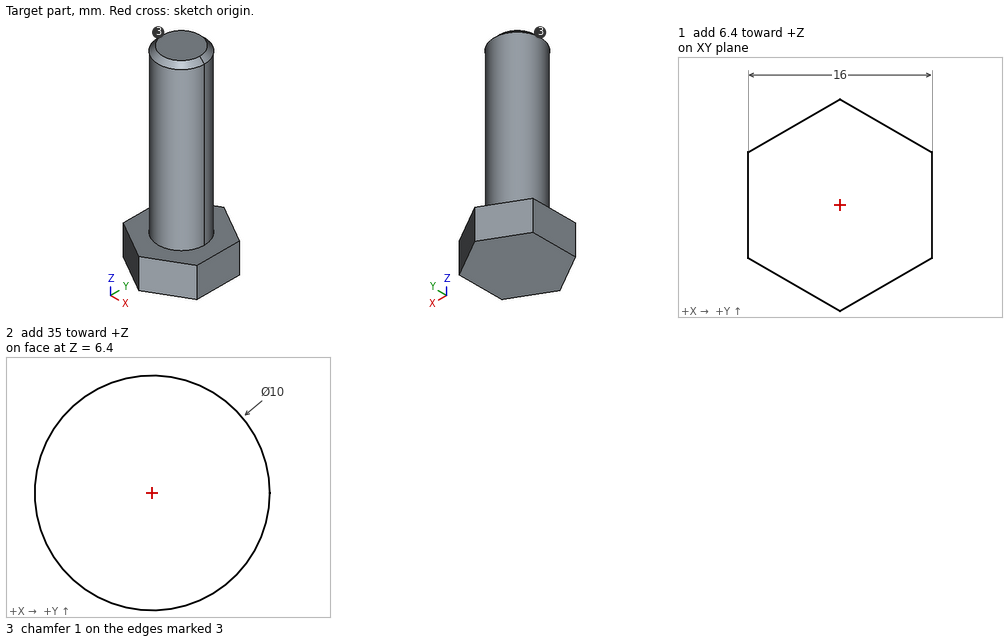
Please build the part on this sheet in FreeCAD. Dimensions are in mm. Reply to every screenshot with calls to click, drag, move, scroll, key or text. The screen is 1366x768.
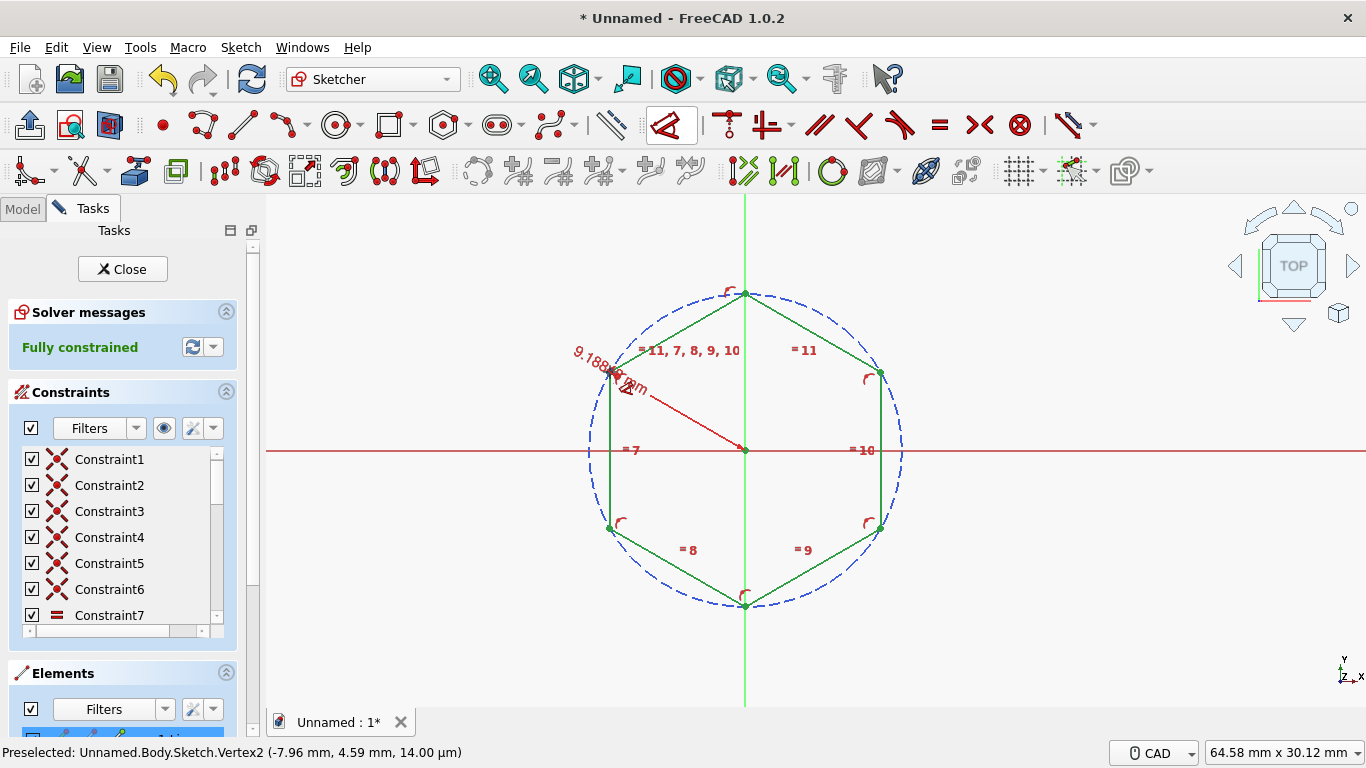
click(881, 529)
click(683, 611)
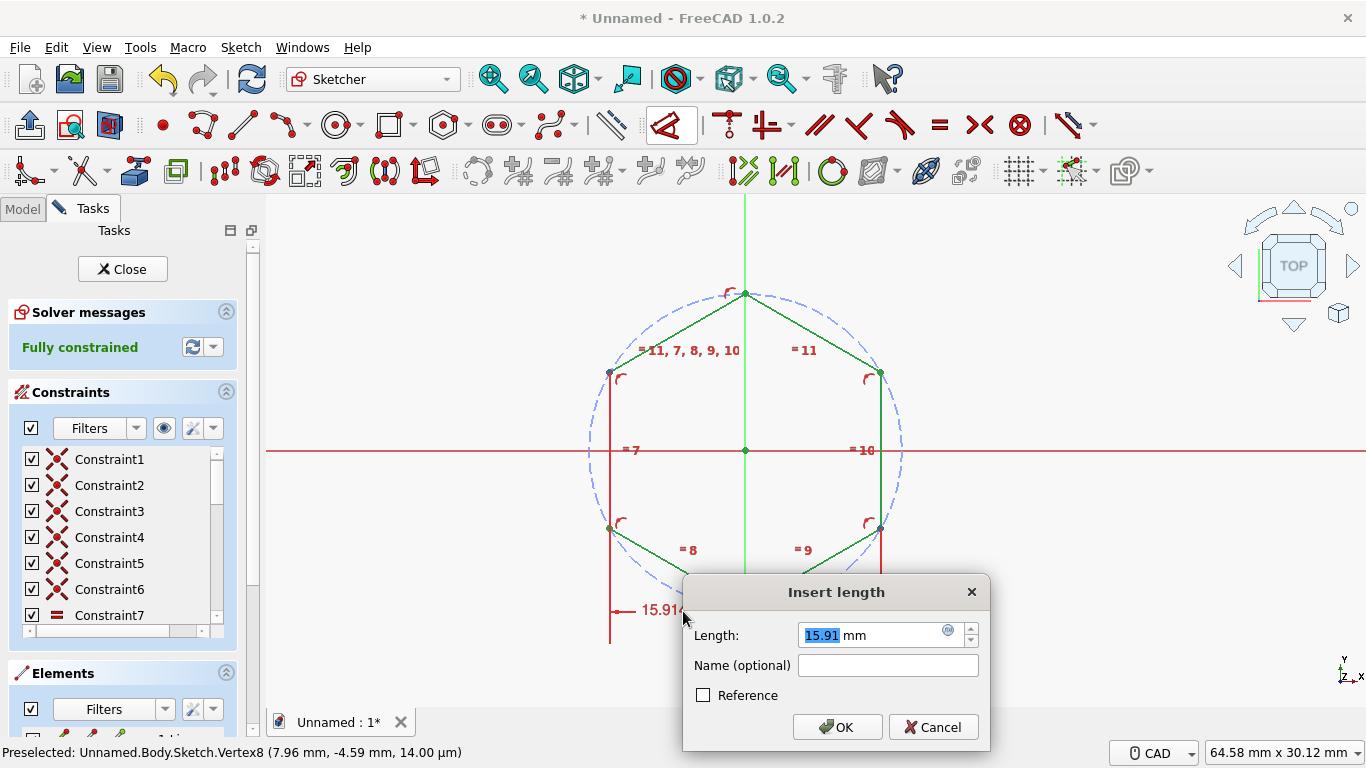
text(16)
key(Return)
key(Escape)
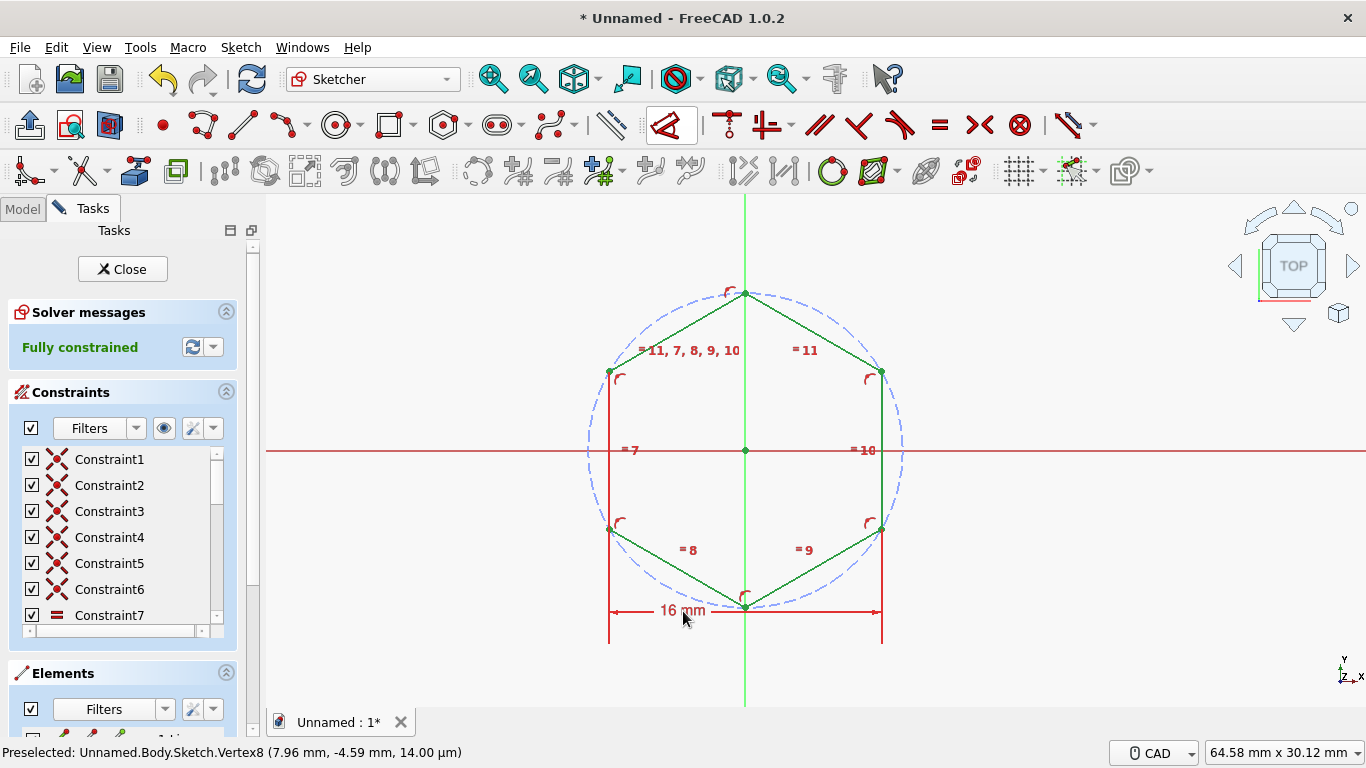
click(123, 269)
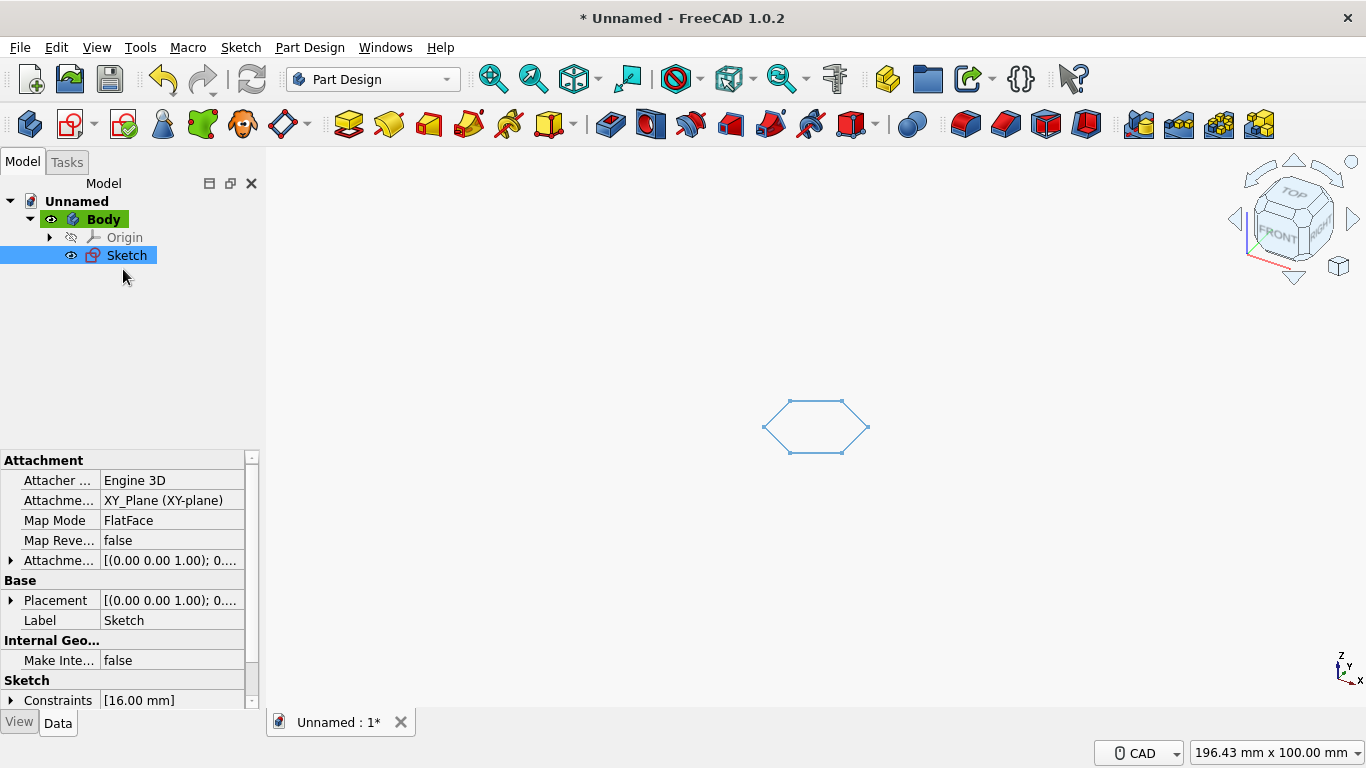
click(350, 124)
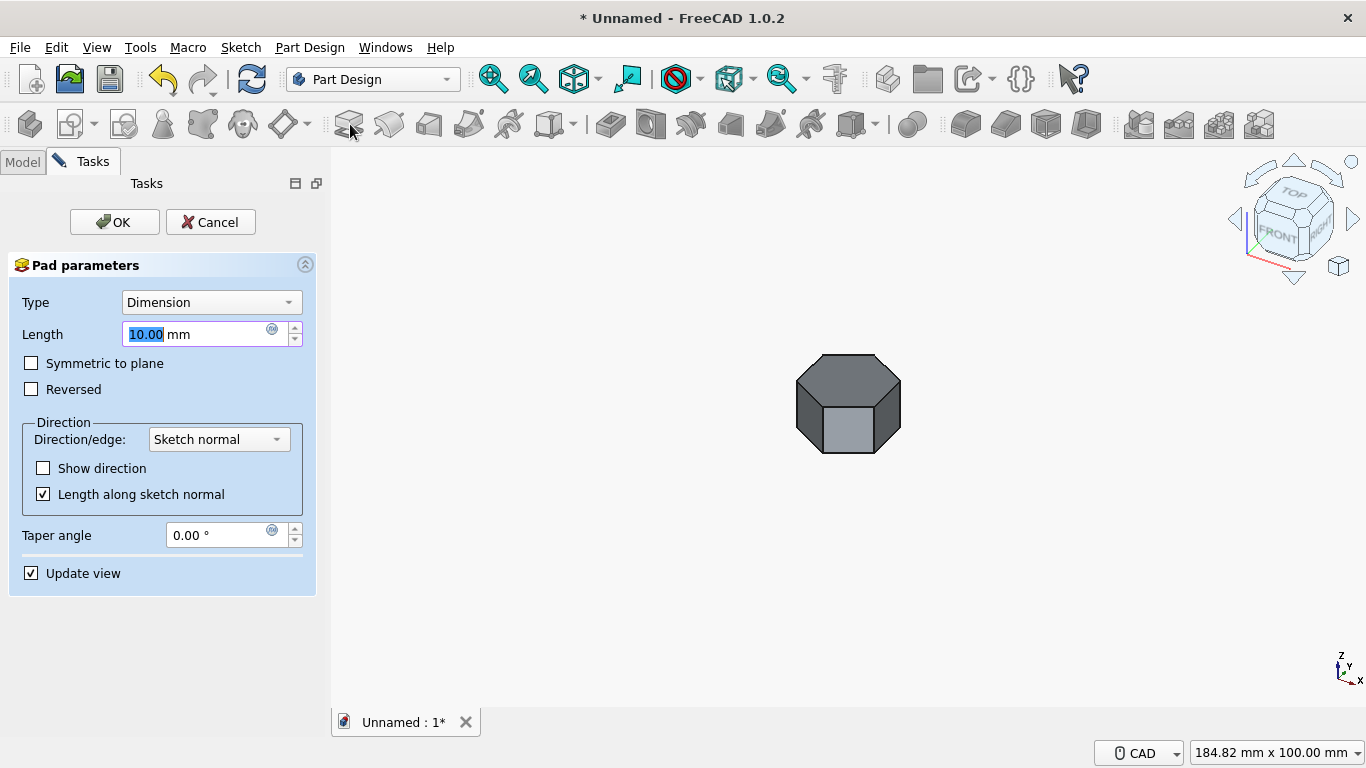
text(6.4)
key(Tab)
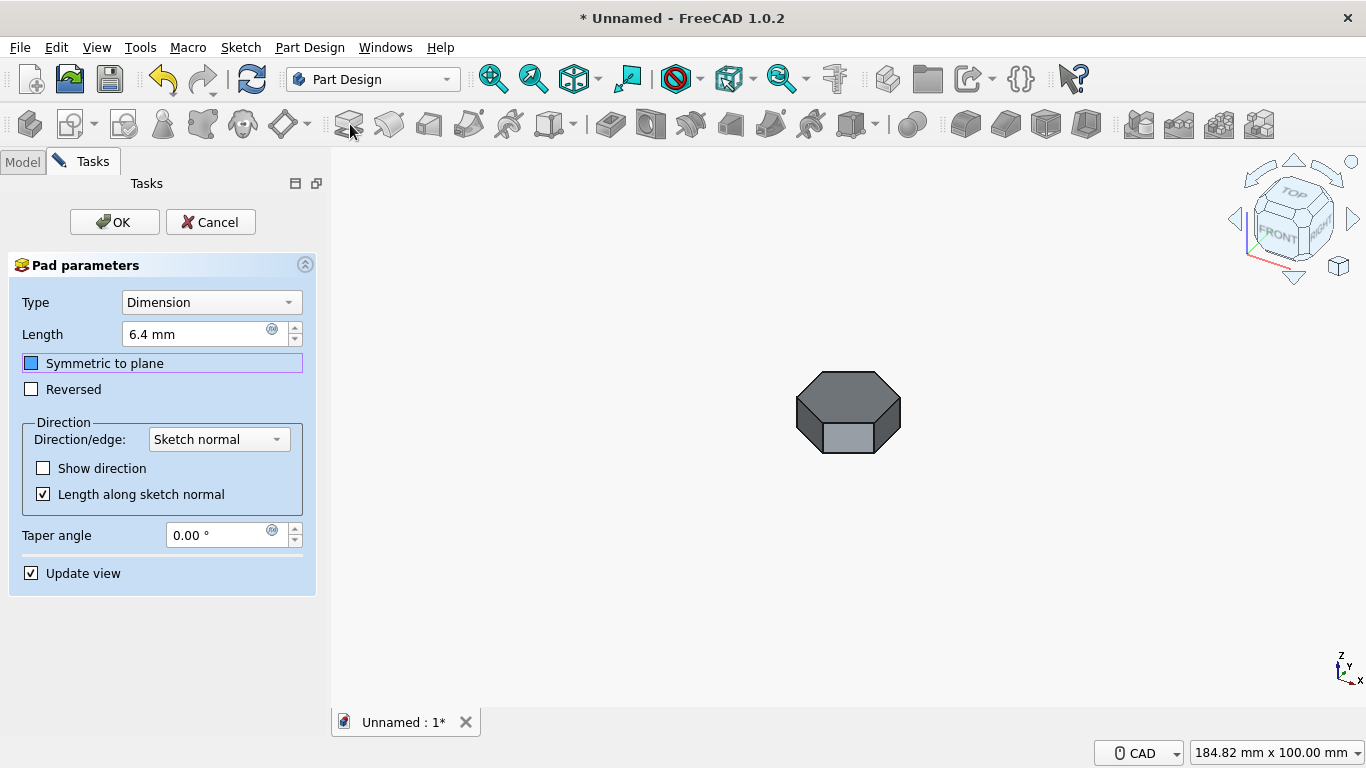
click(115, 222)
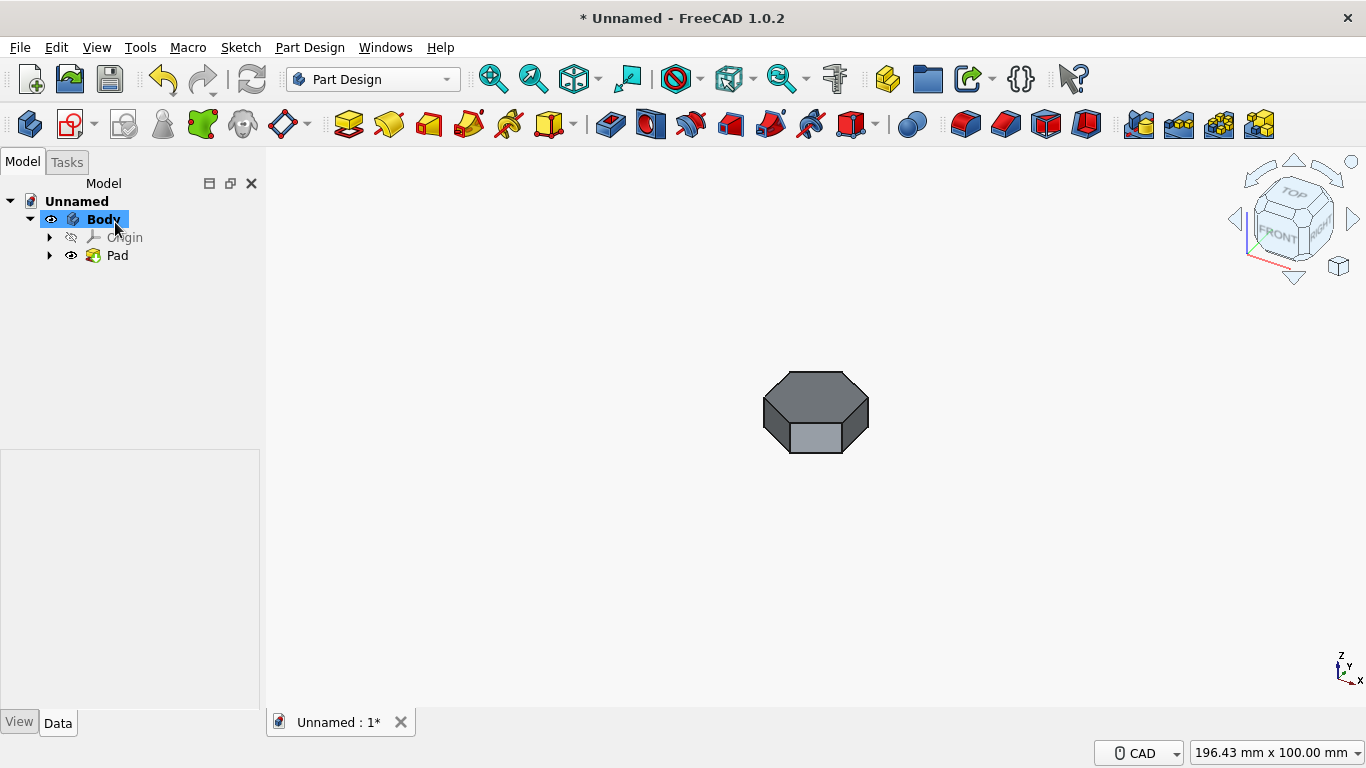
key(v)
key(f)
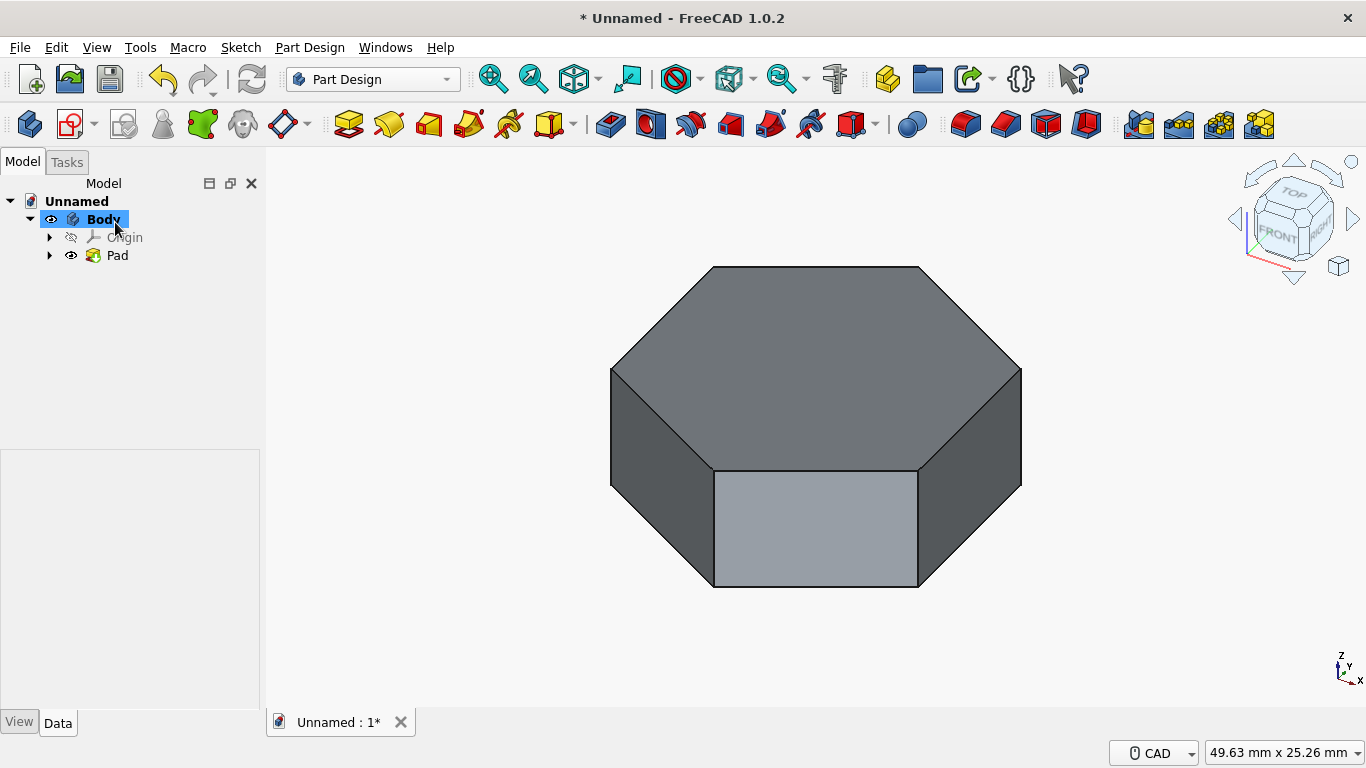
click(816, 368)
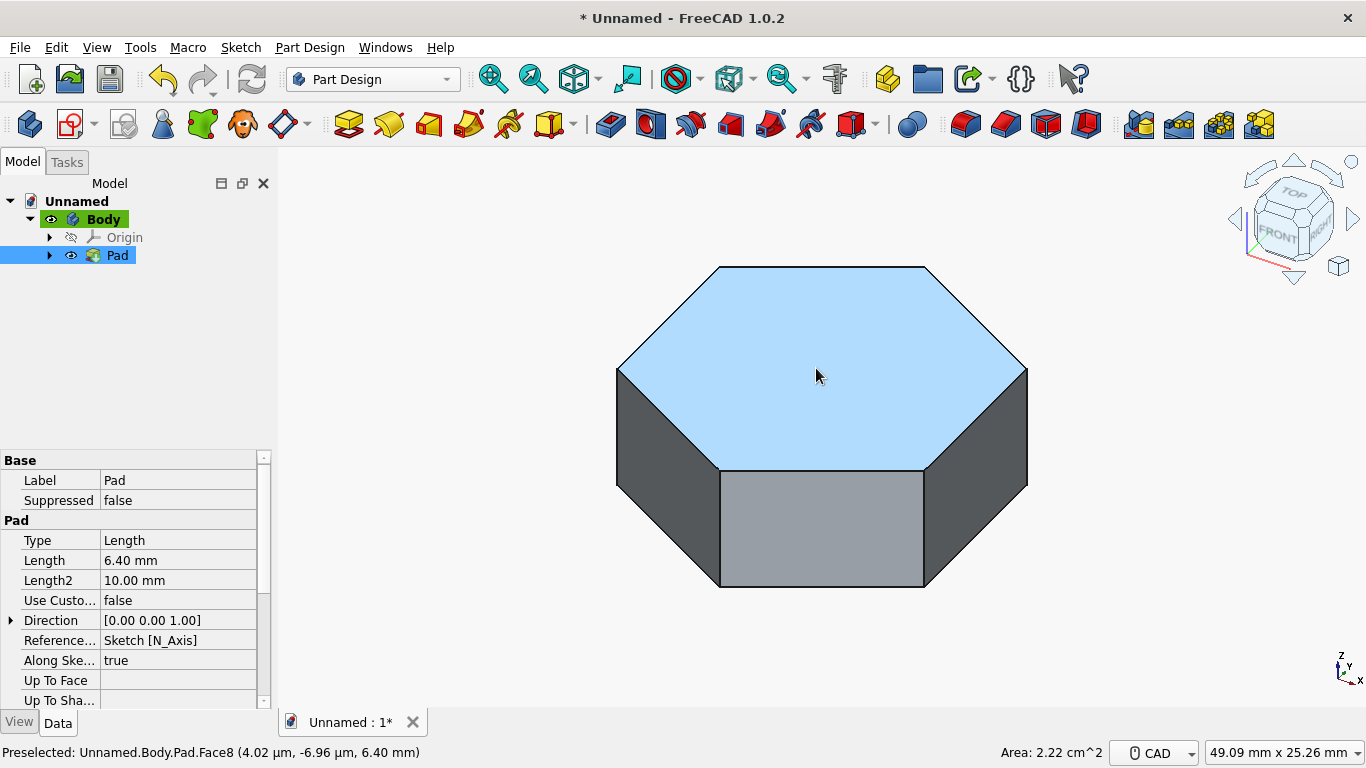
click(70, 124)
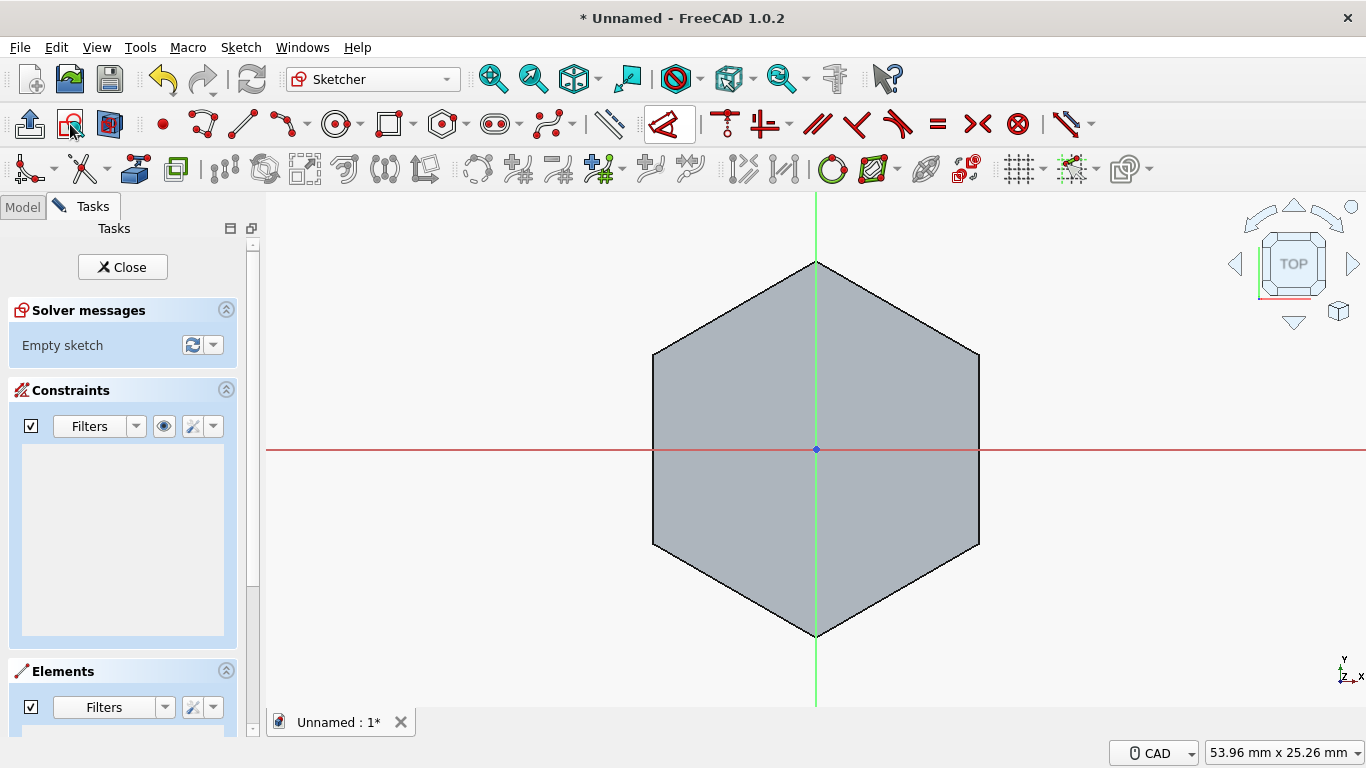
scroll(955, 450, up, 2)